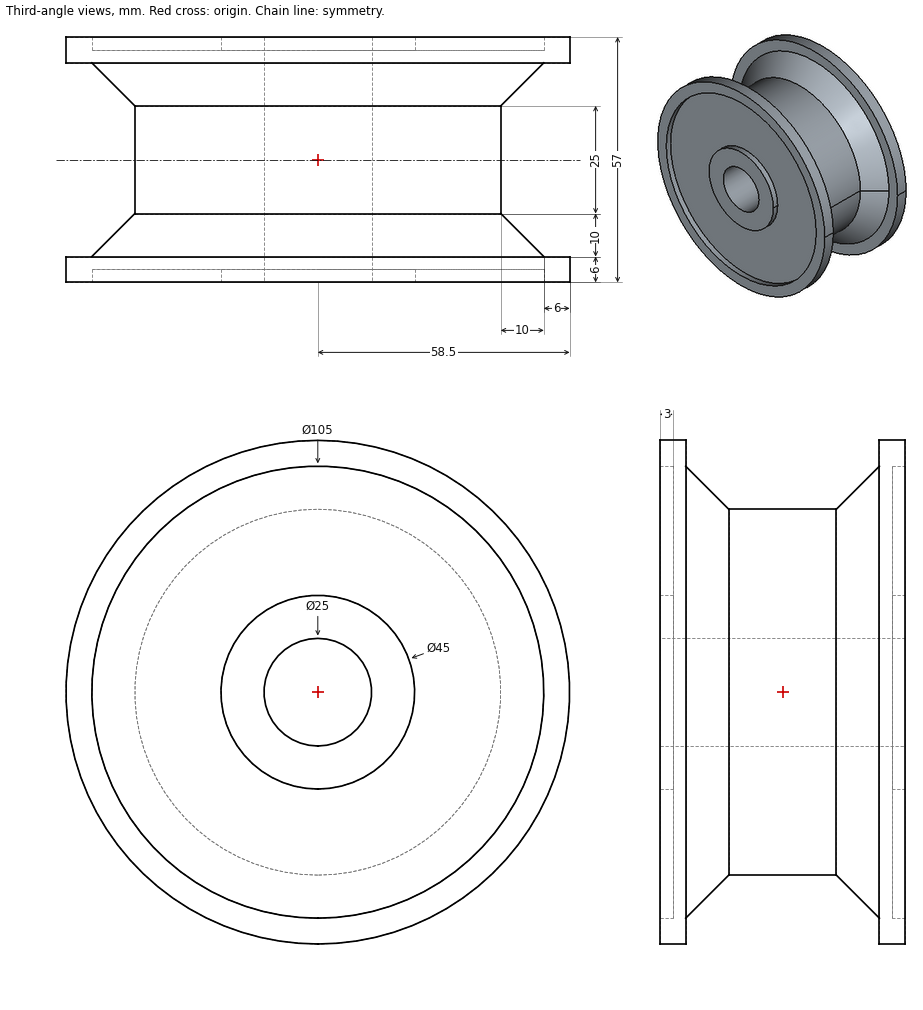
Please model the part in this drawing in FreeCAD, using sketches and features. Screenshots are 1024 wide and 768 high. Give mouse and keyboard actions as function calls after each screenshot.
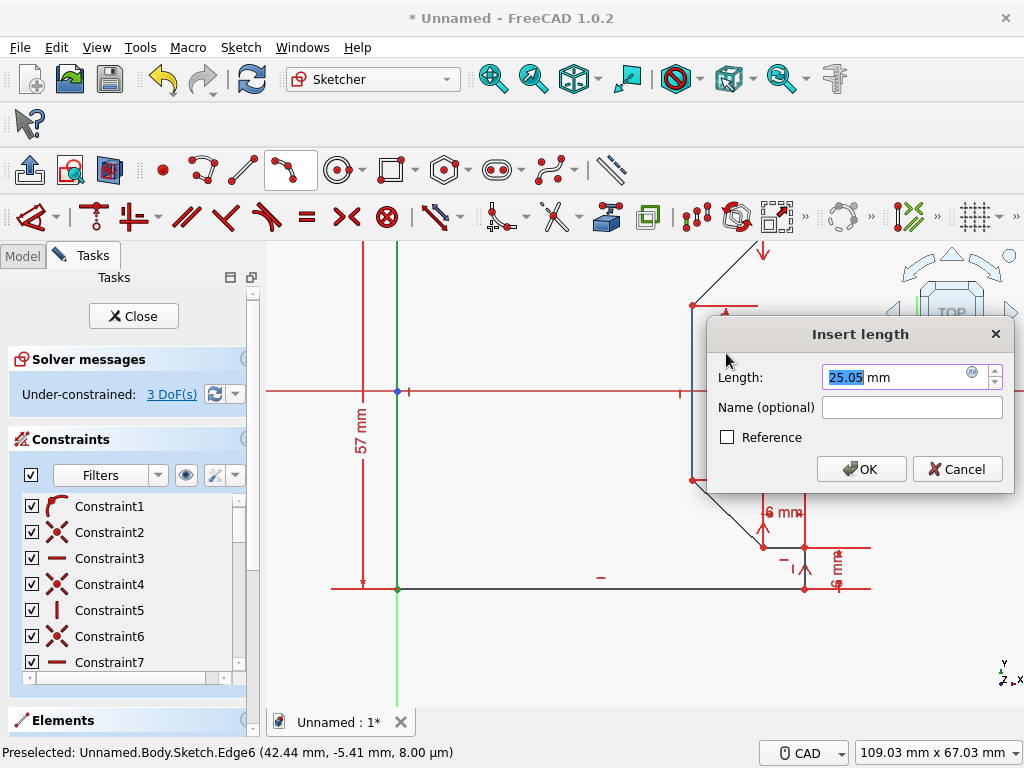
text(25)
key(Return)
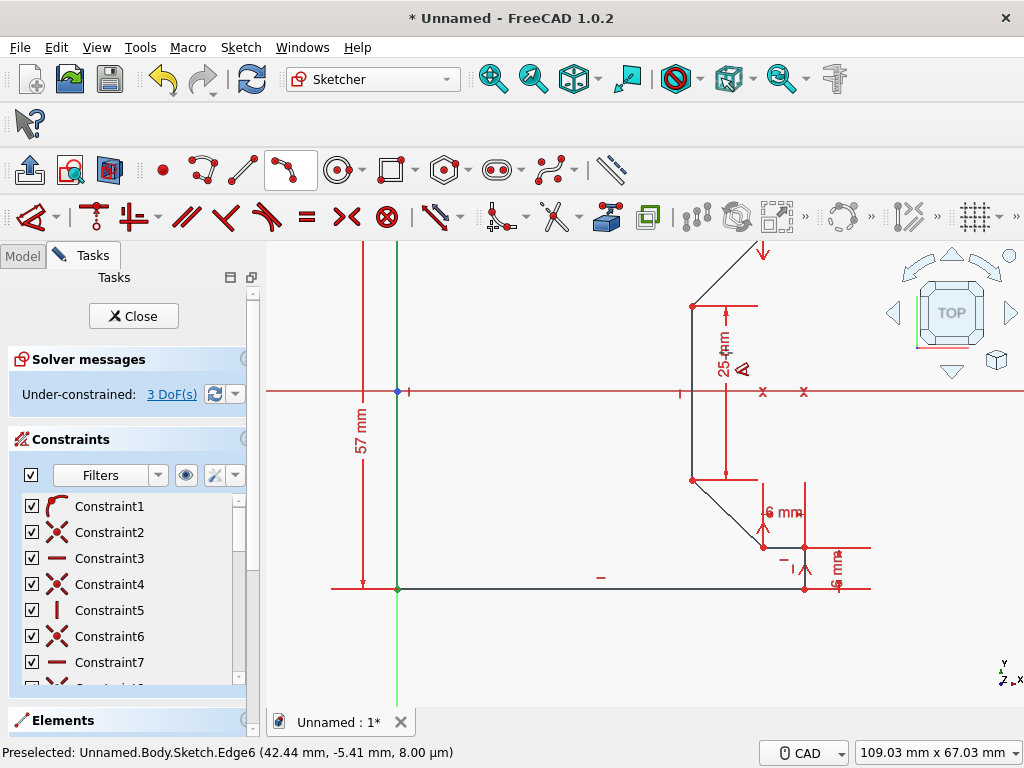
click(742, 527)
click(728, 446)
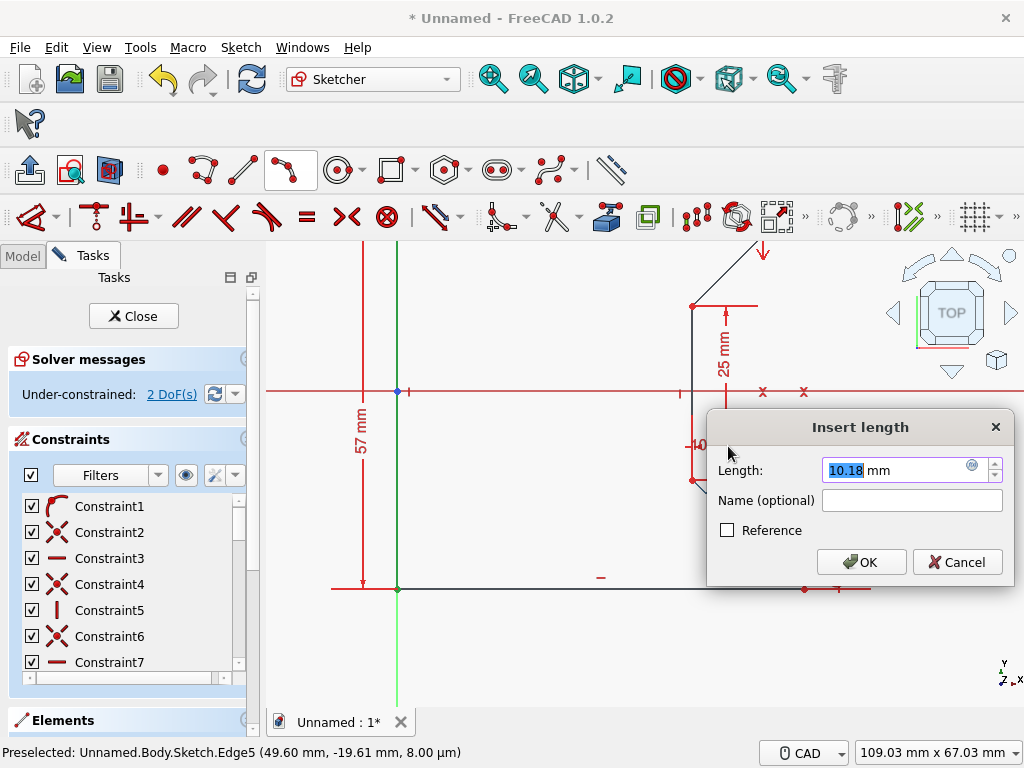
text(10)
key(Return)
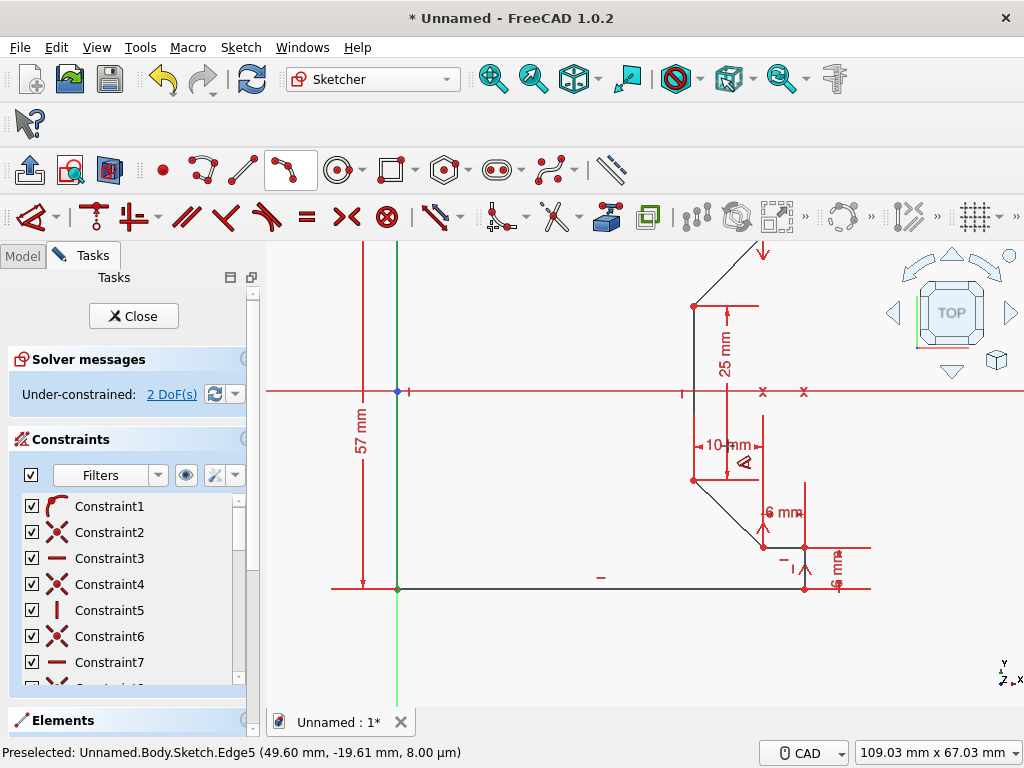
click(742, 527)
click(797, 490)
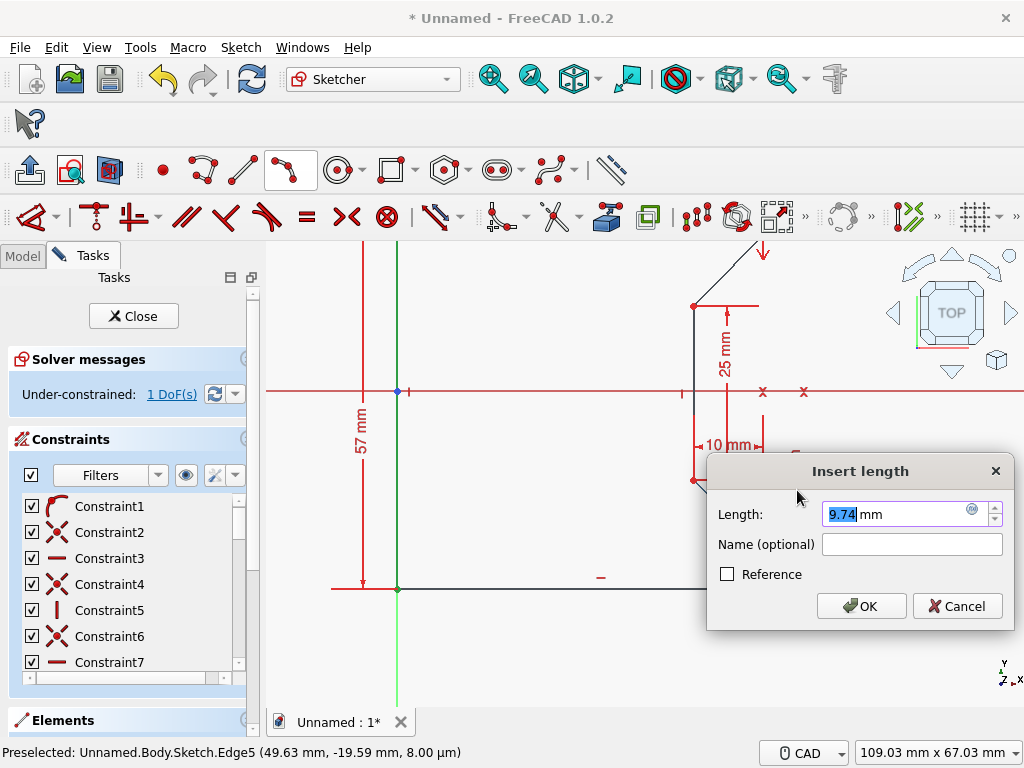
text(10)
key(Return)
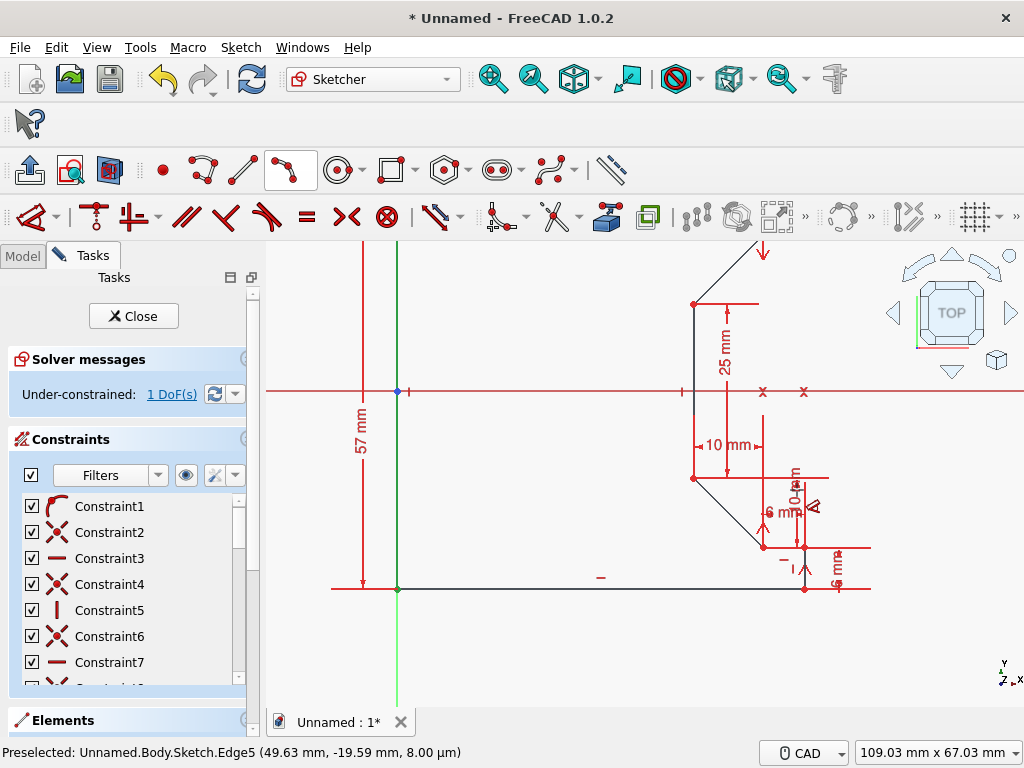
click(520, 589)
click(601, 623)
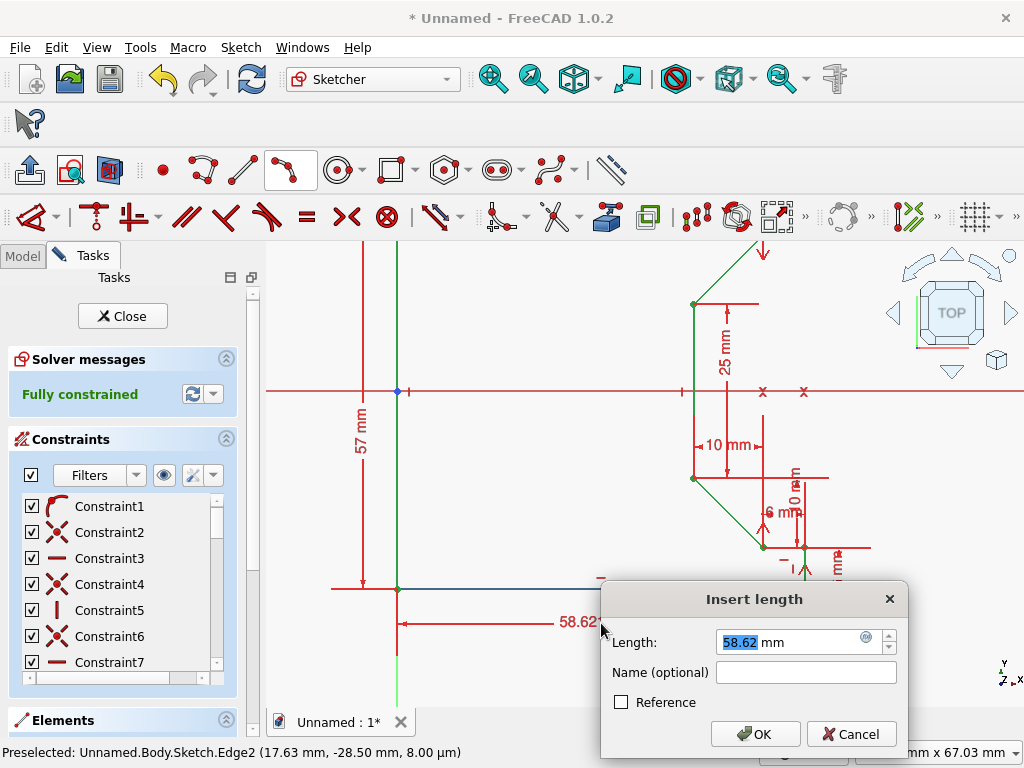
text(58.5)
key(Return)
key(Escape)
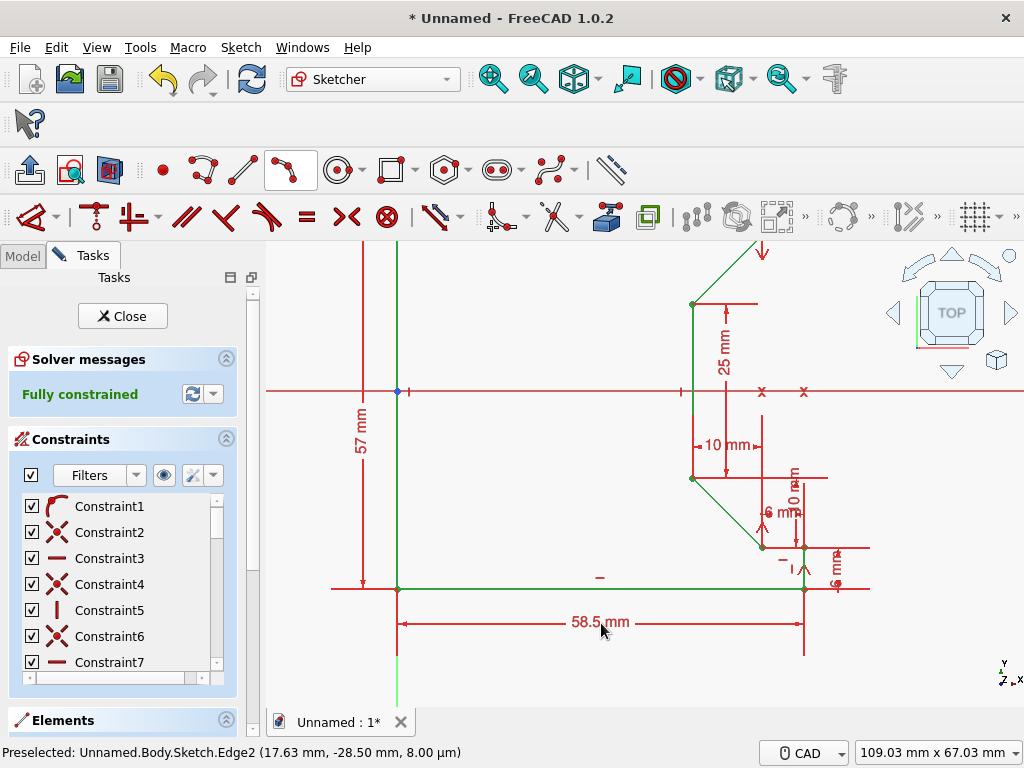
click(123, 316)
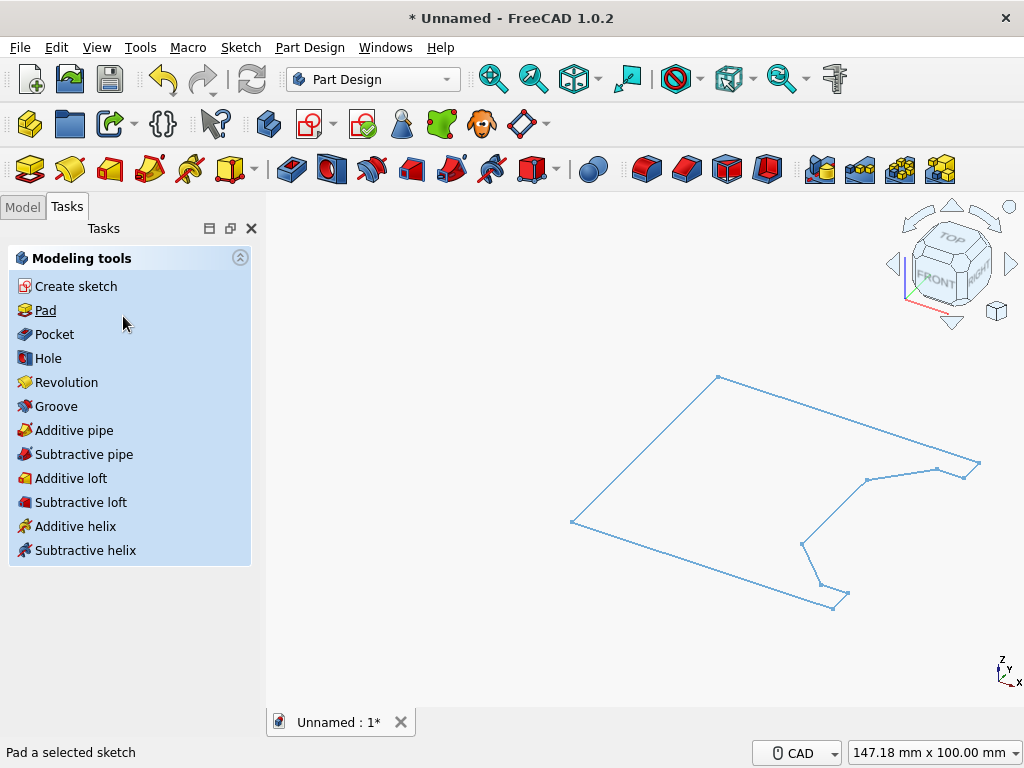
click(70, 170)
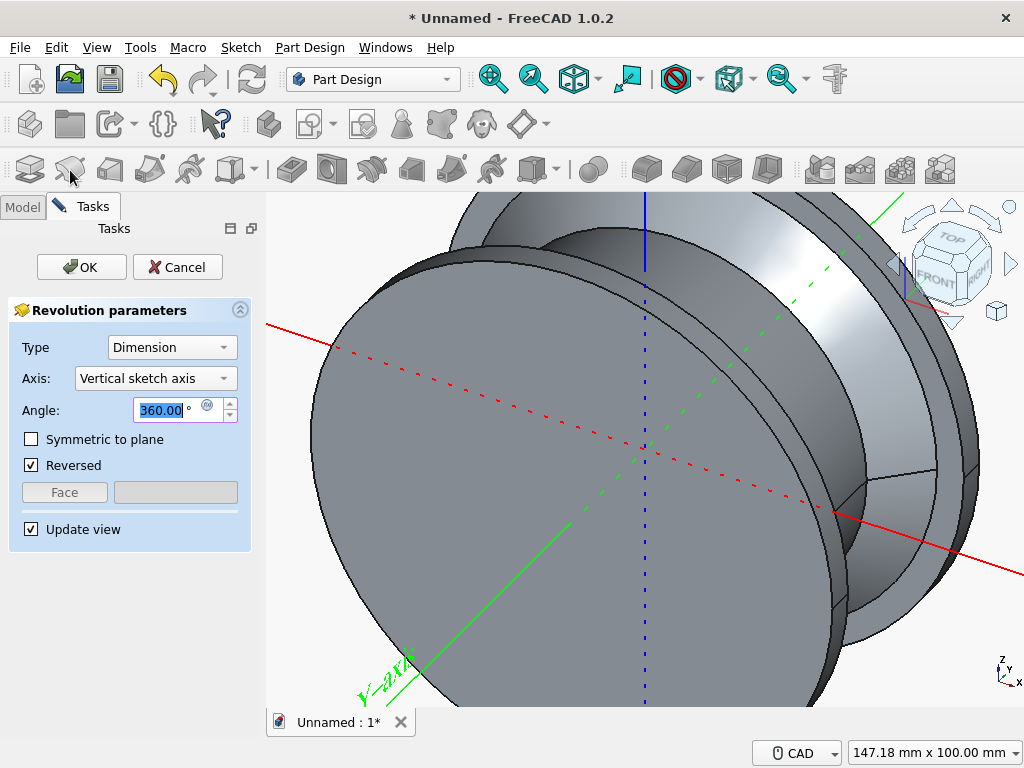
click(82, 267)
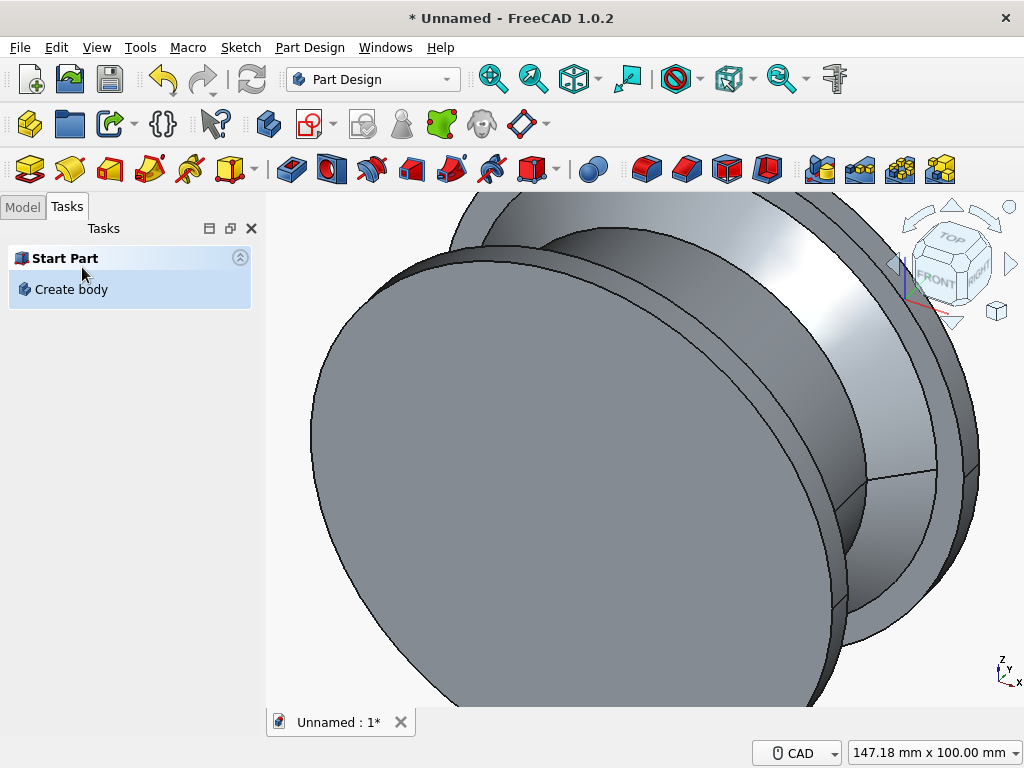
click(494, 80)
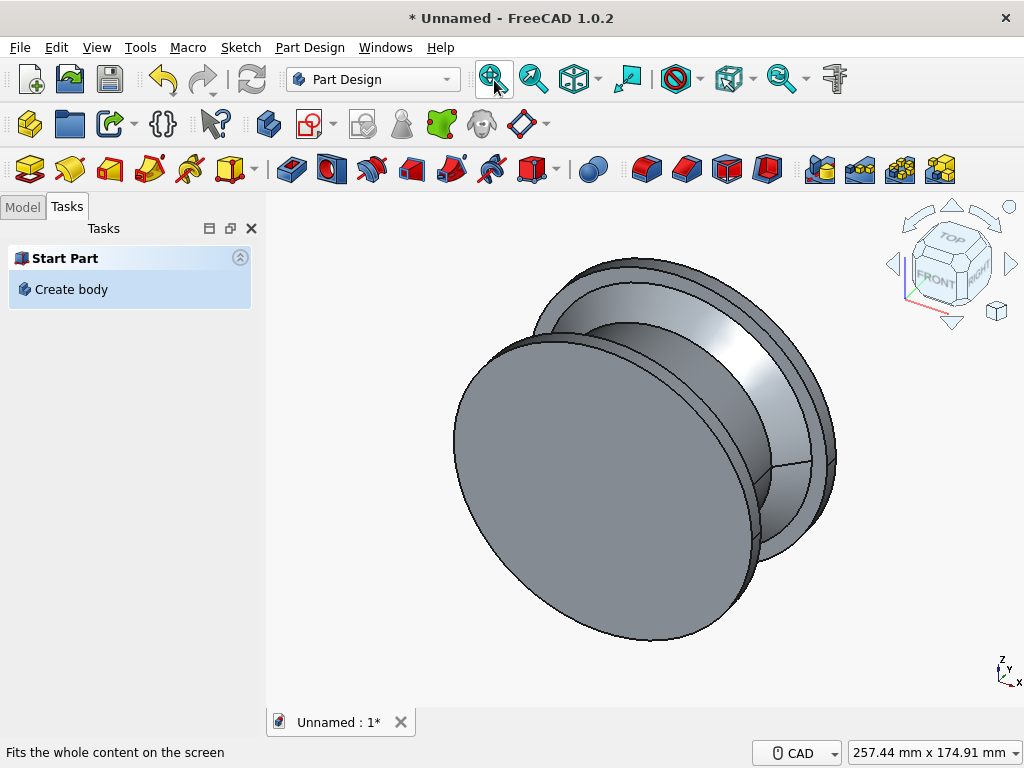
click(603, 490)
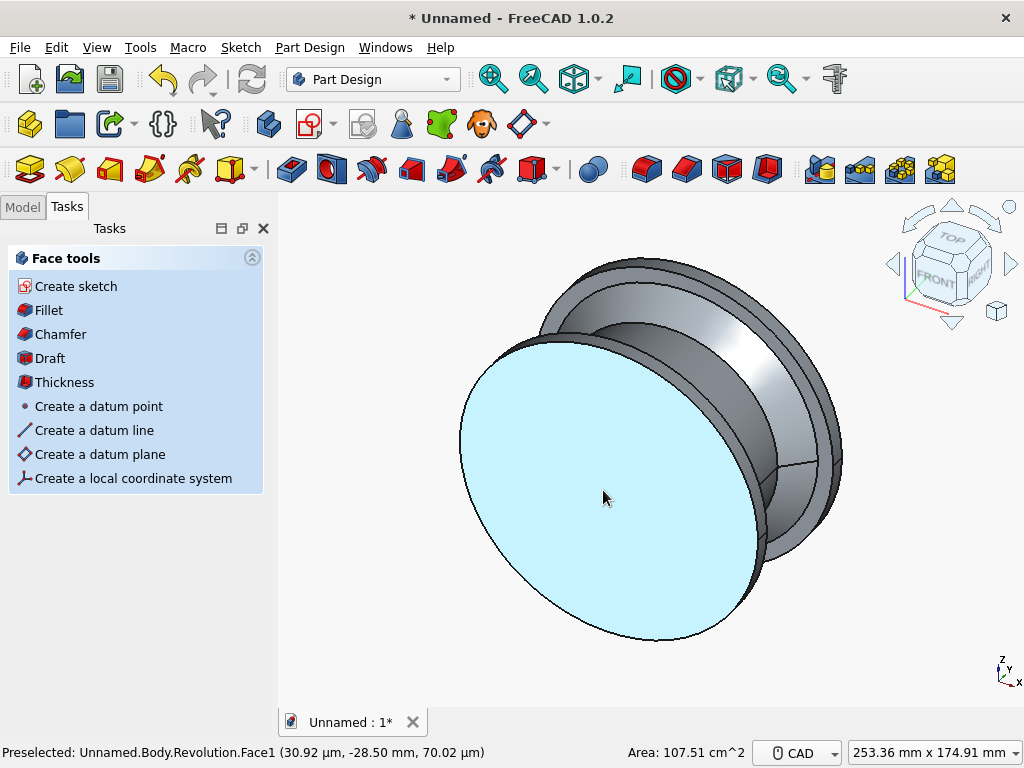
click(310, 124)